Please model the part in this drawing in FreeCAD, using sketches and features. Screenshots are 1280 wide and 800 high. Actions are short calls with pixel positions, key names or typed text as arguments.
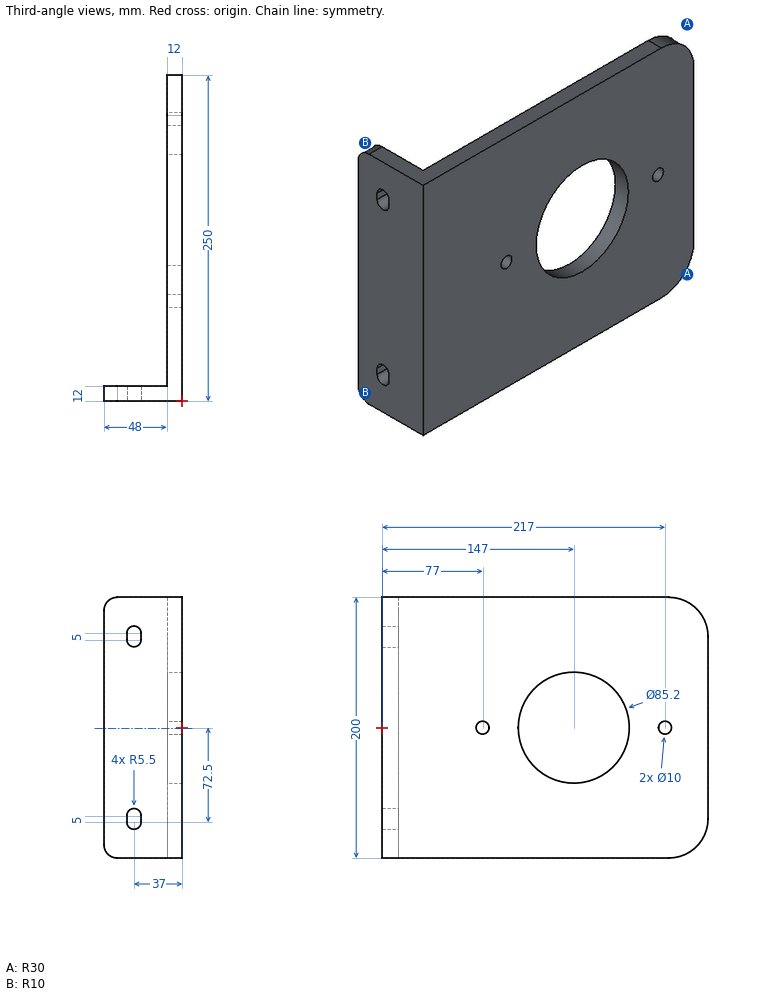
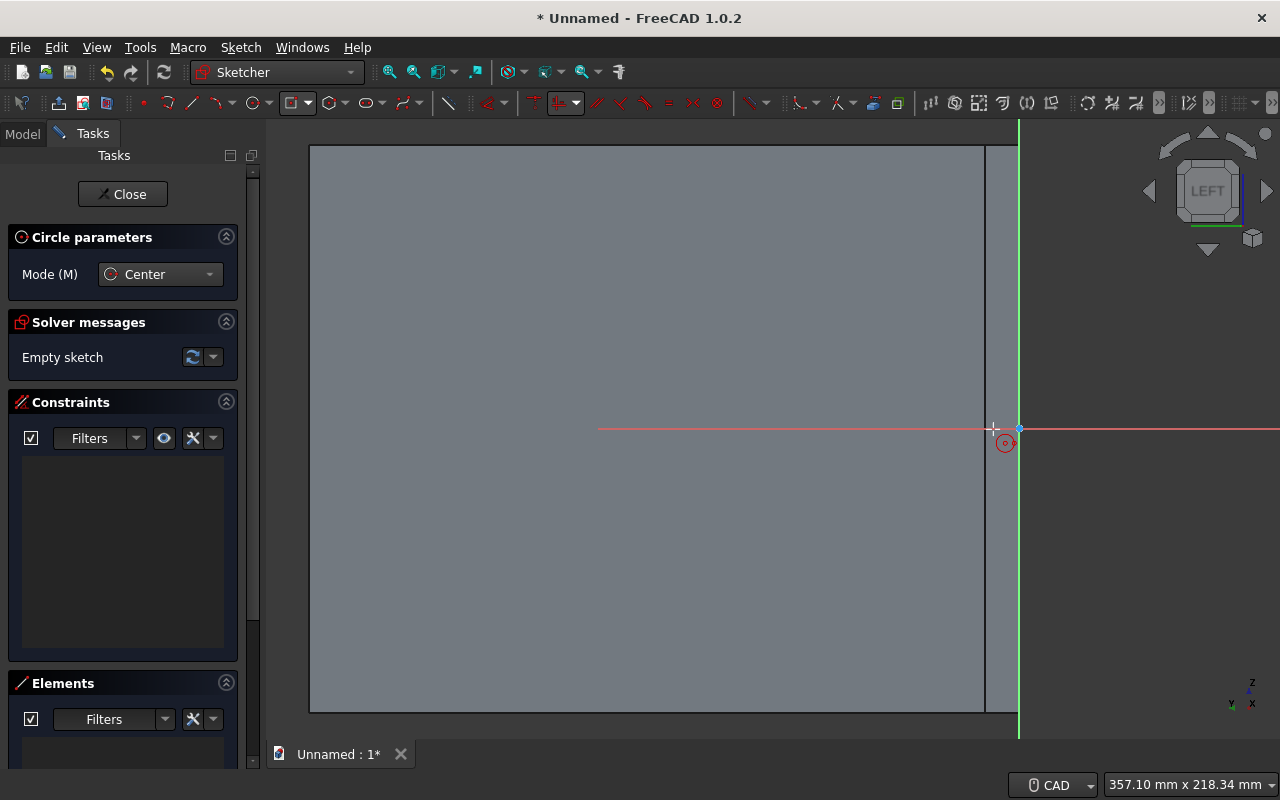
click(602, 429)
move(688, 343)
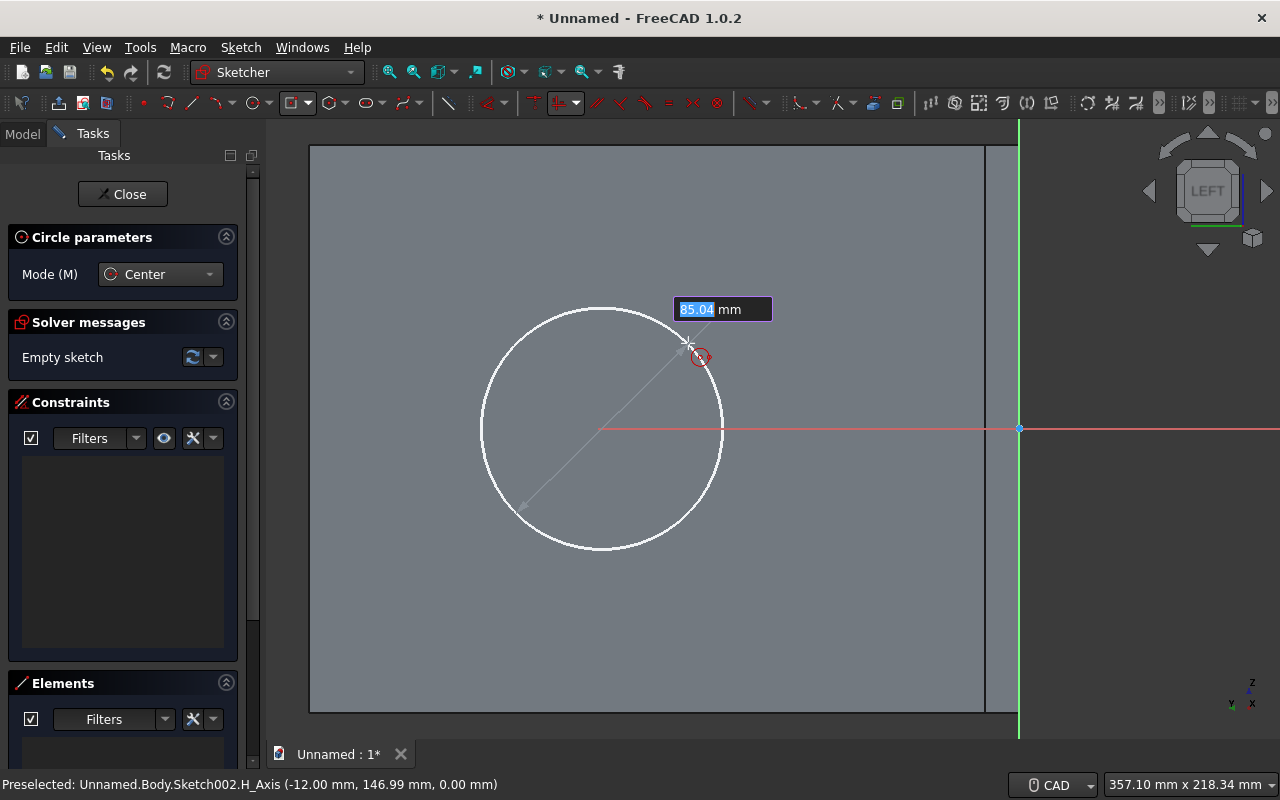
text(85.2)
key(Return)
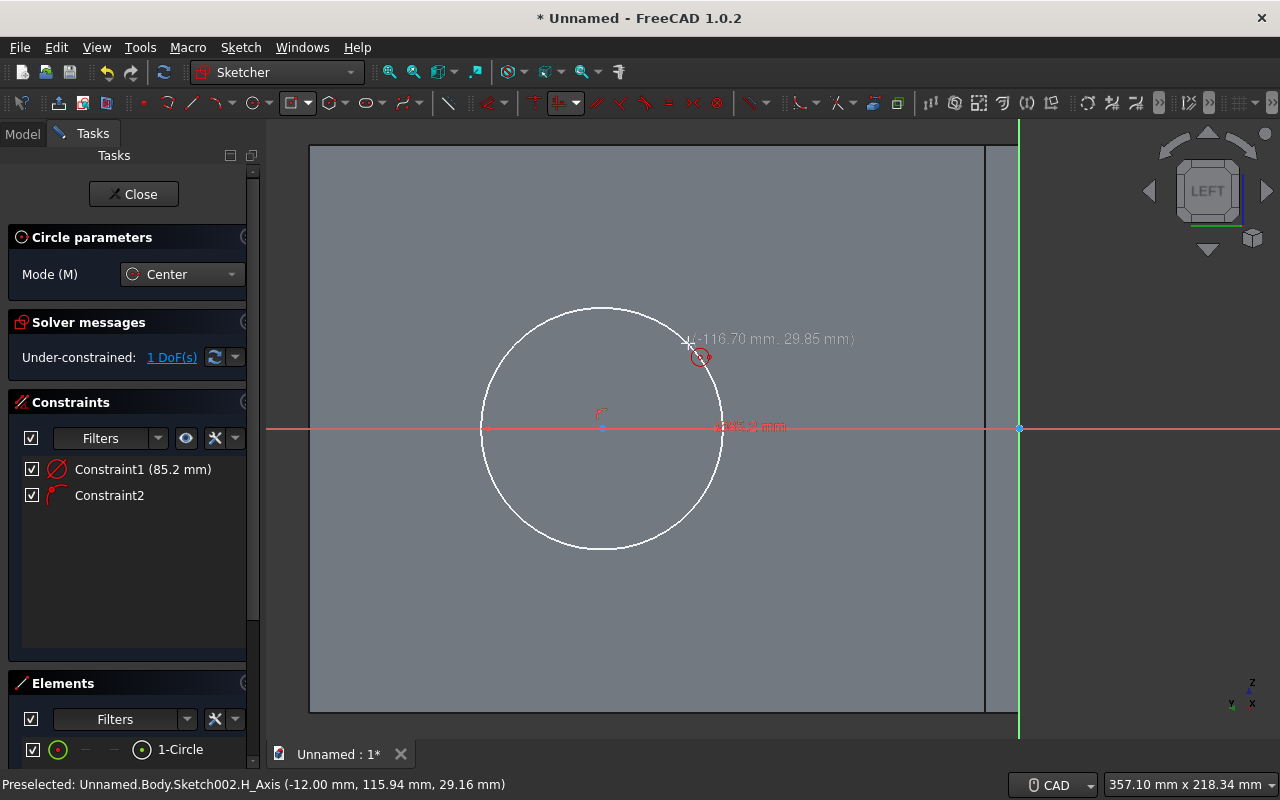
scroll(403, 429, up, 3)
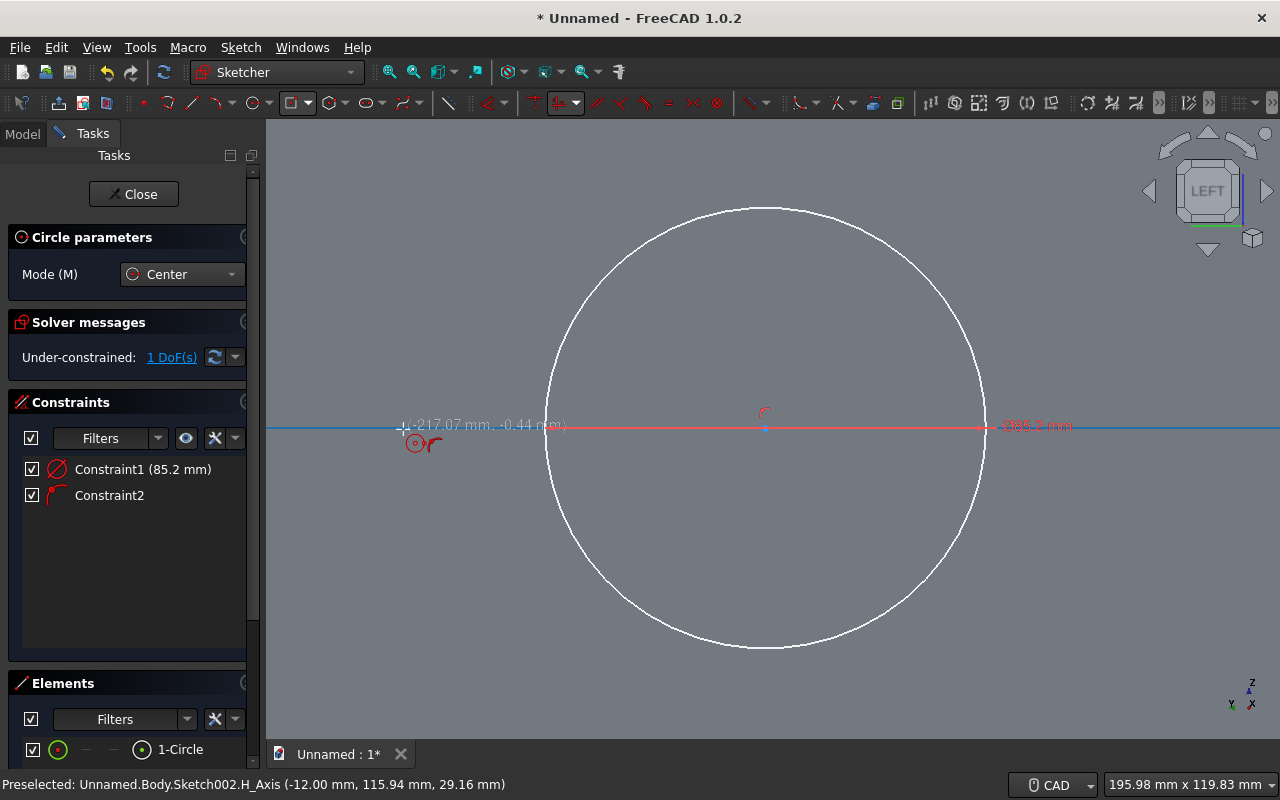
click(403, 428)
move(422, 410)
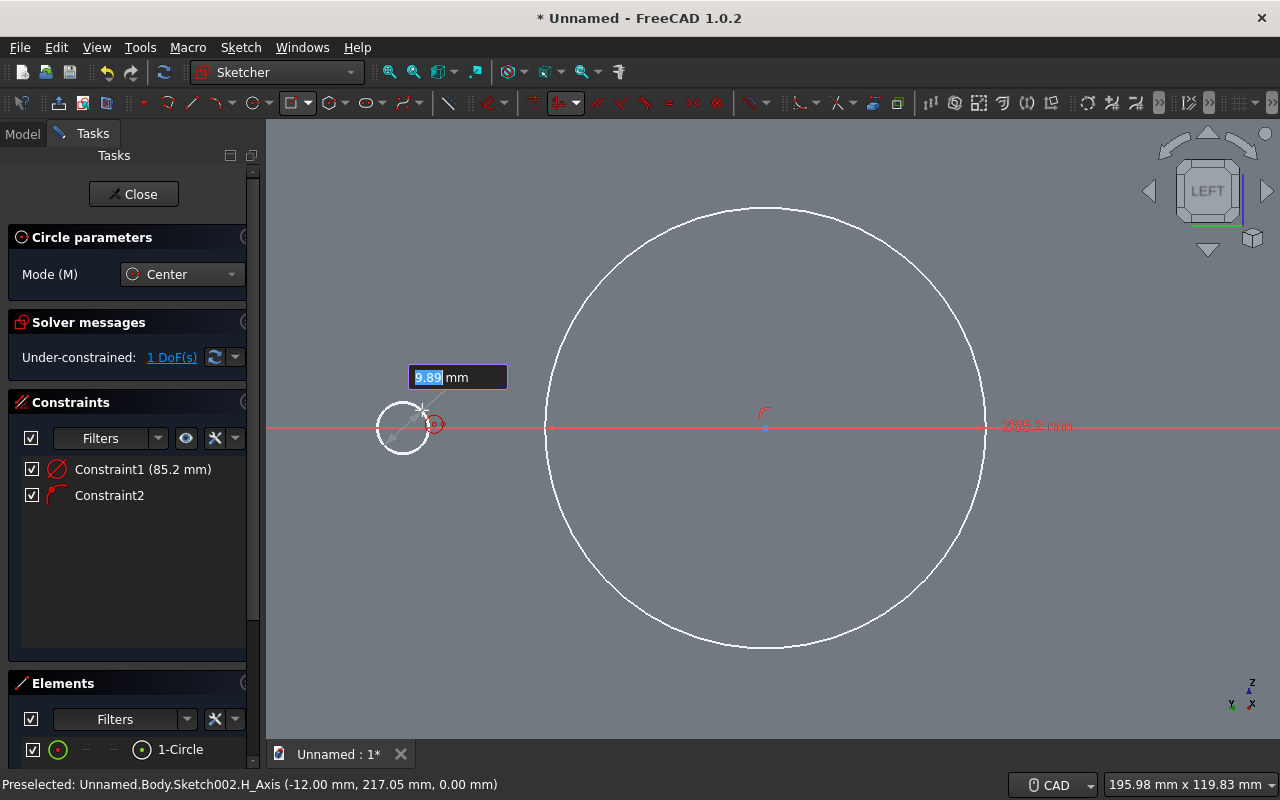
text(10)
key(Return)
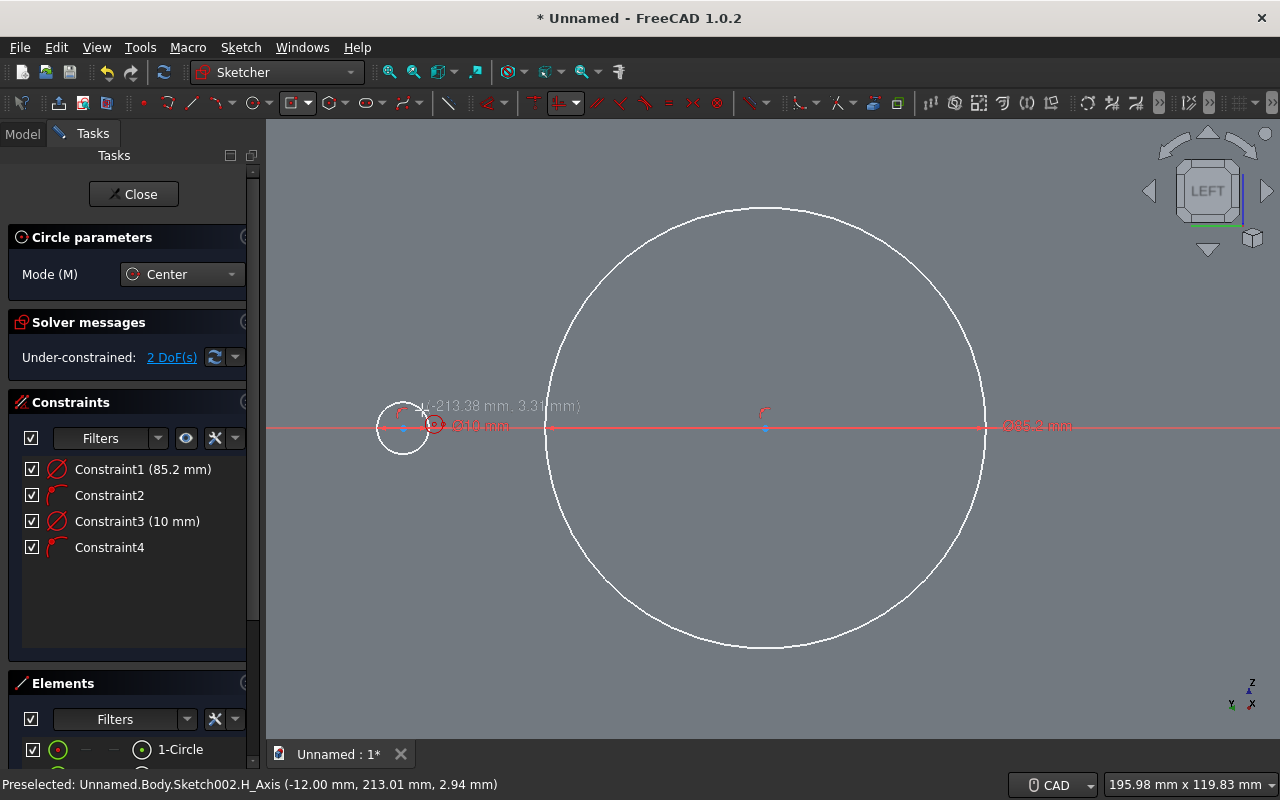
scroll(404, 430, down, 3)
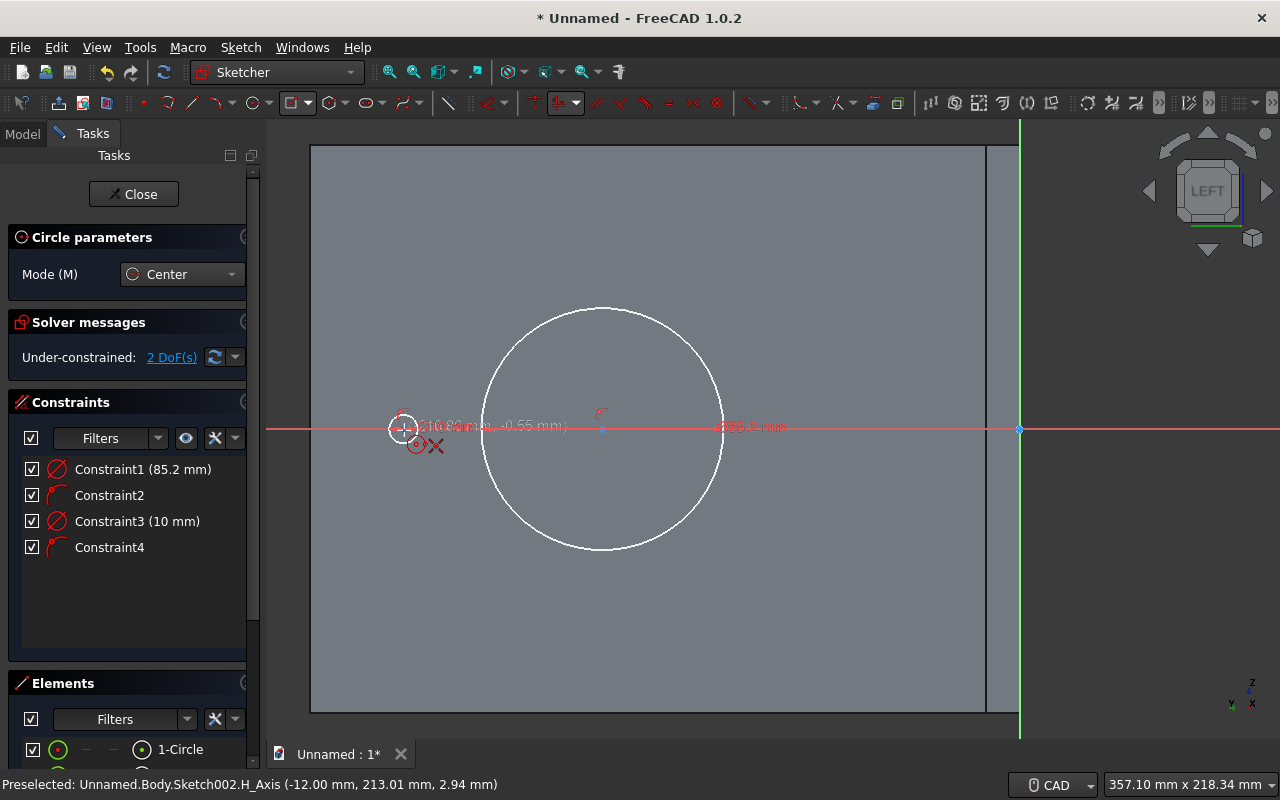
scroll(801, 429, up, 3)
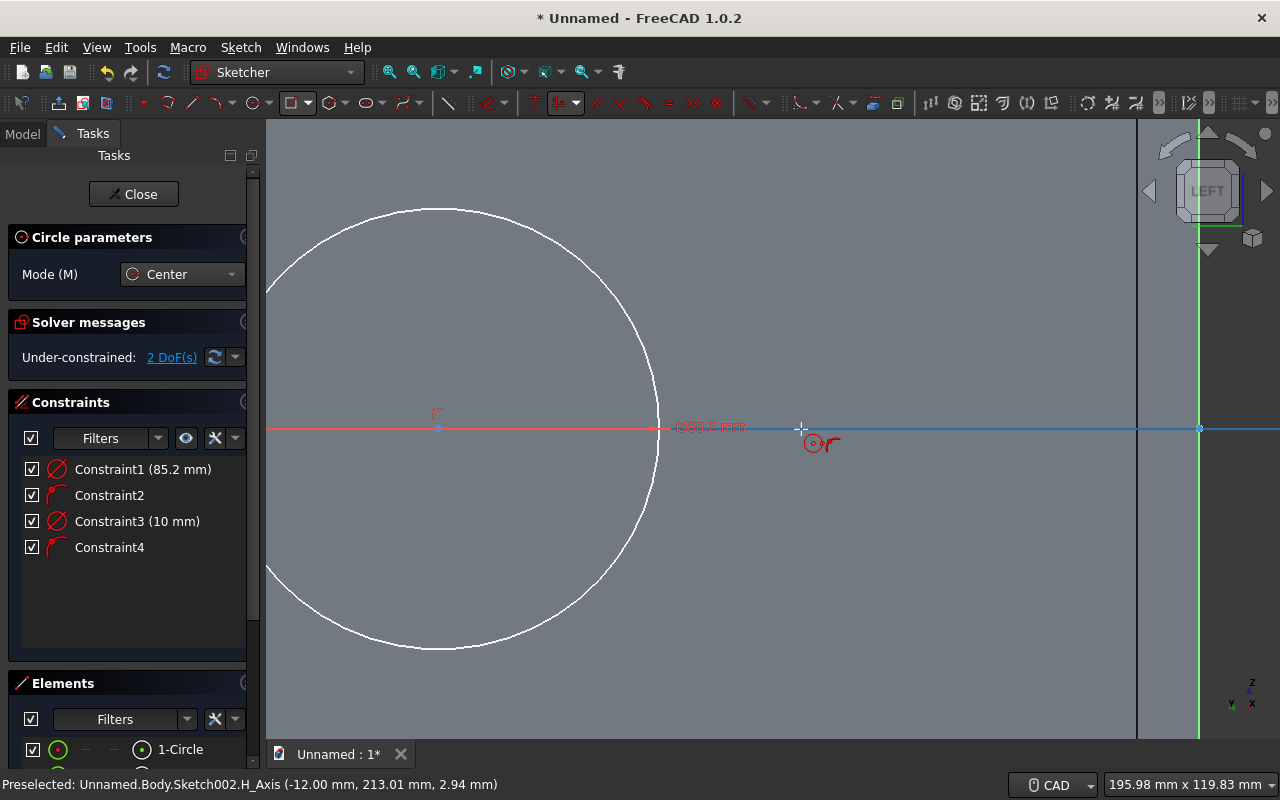
click(801, 429)
move(819, 411)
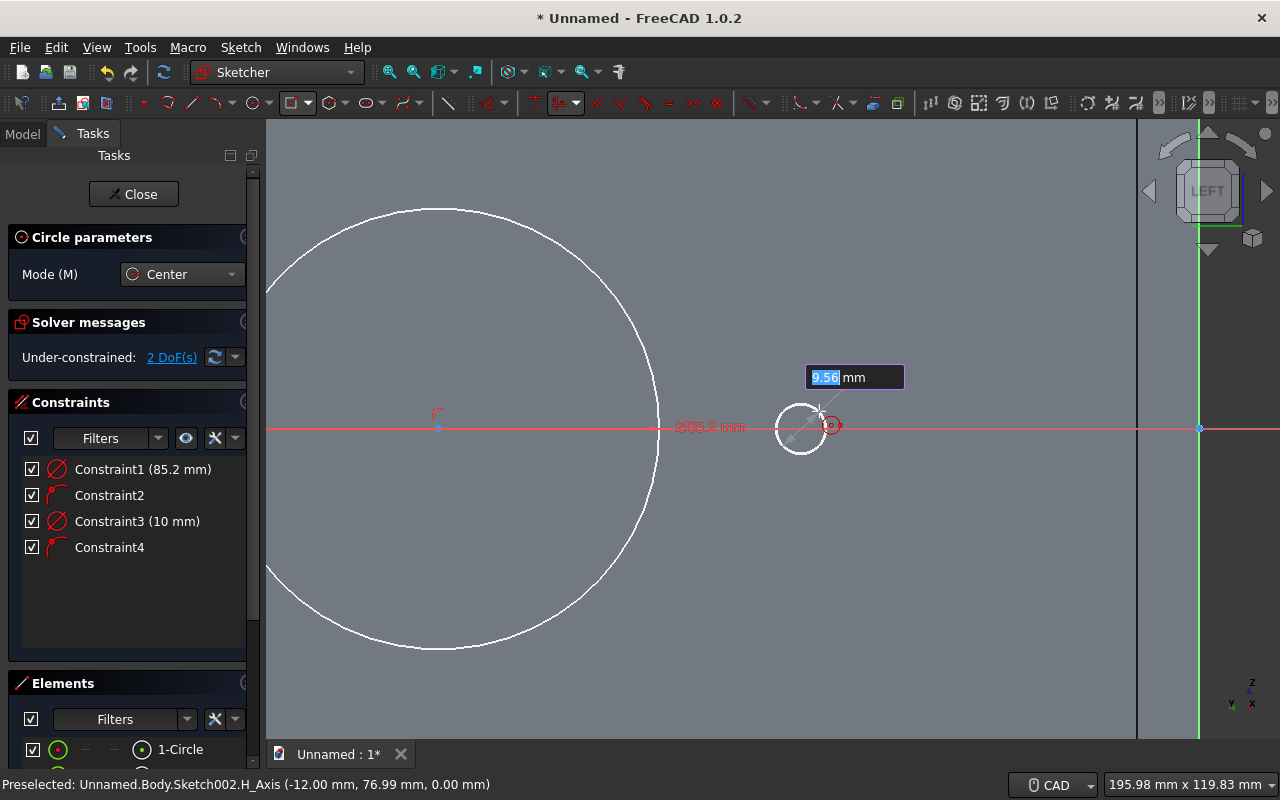
text(10)
key(Return)
key(Escape)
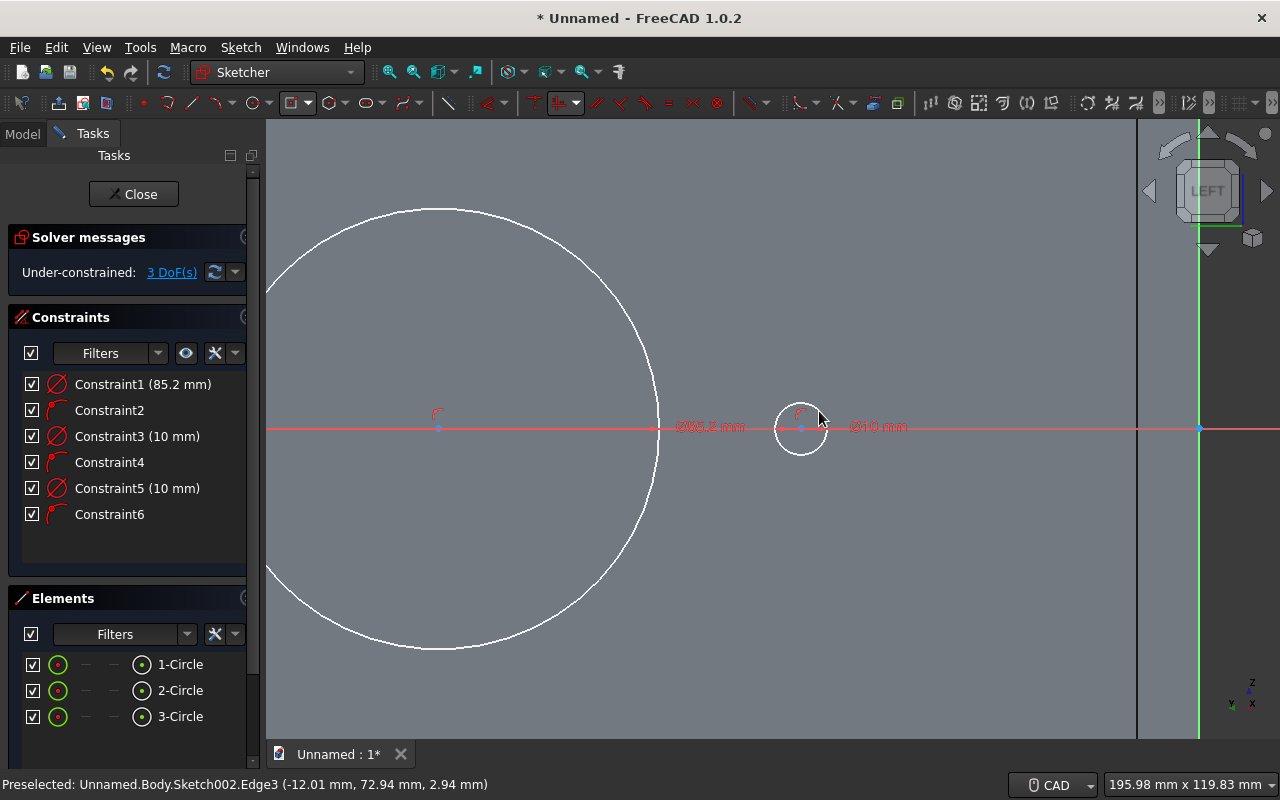
click(488, 104)